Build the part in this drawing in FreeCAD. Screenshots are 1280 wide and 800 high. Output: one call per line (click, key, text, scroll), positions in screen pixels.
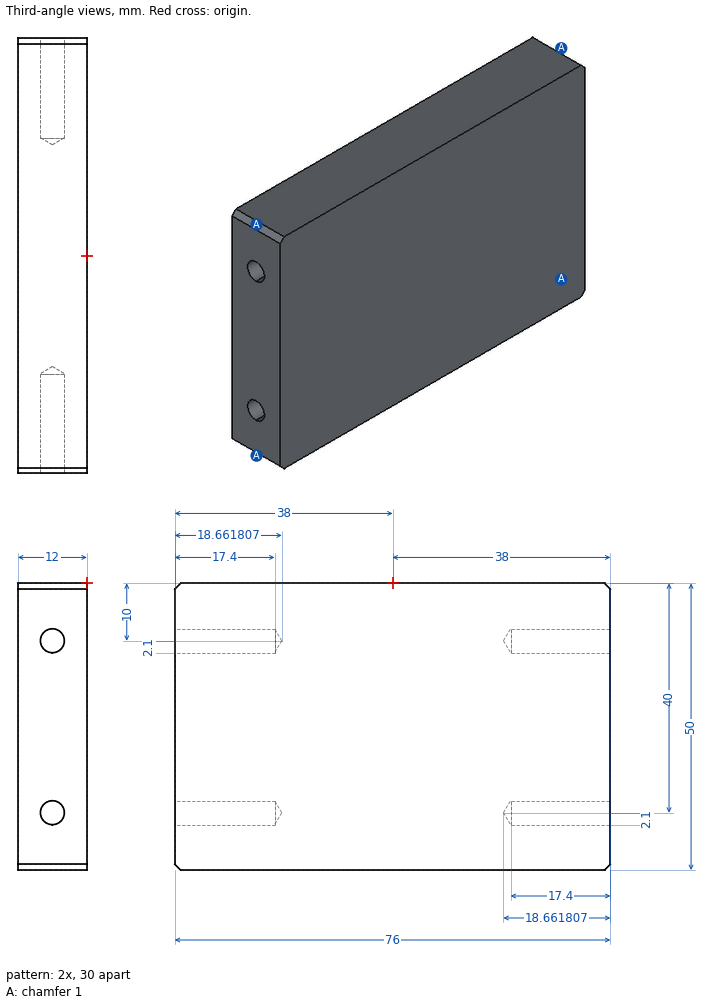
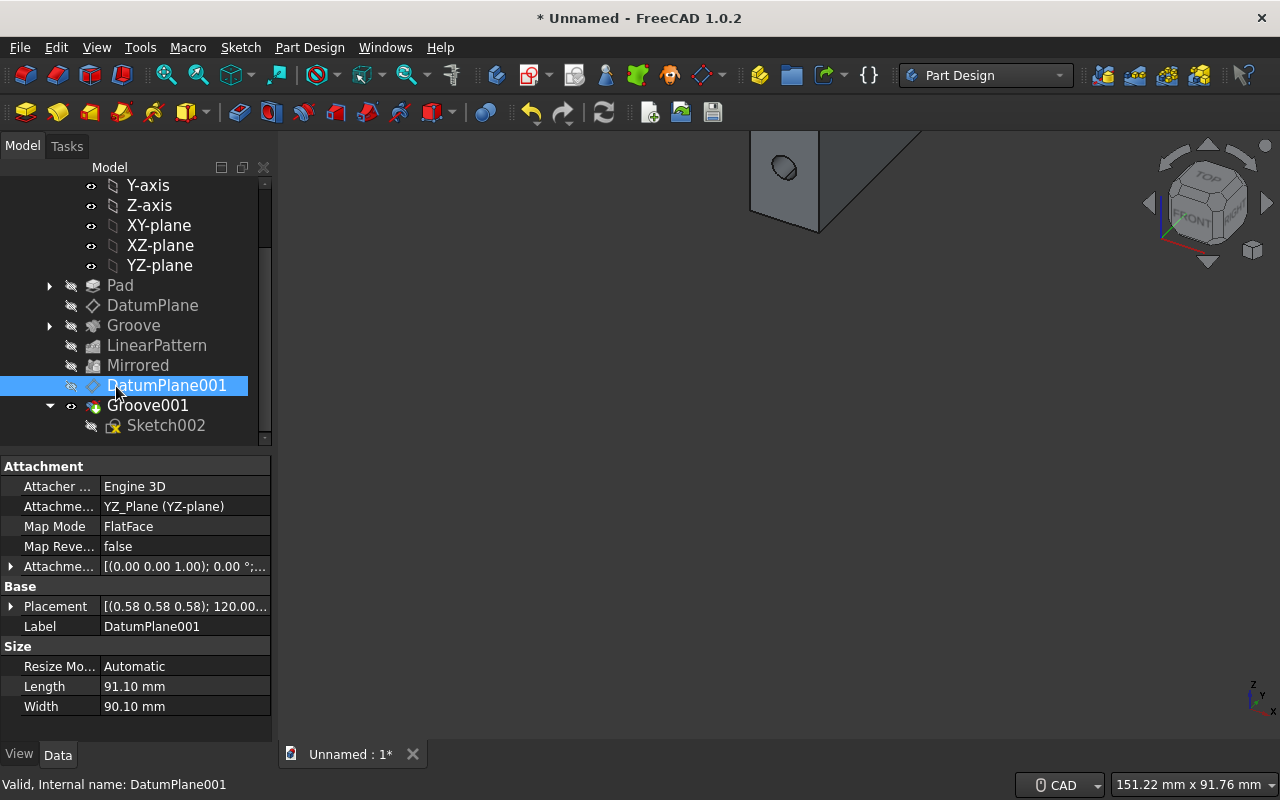
click(168, 76)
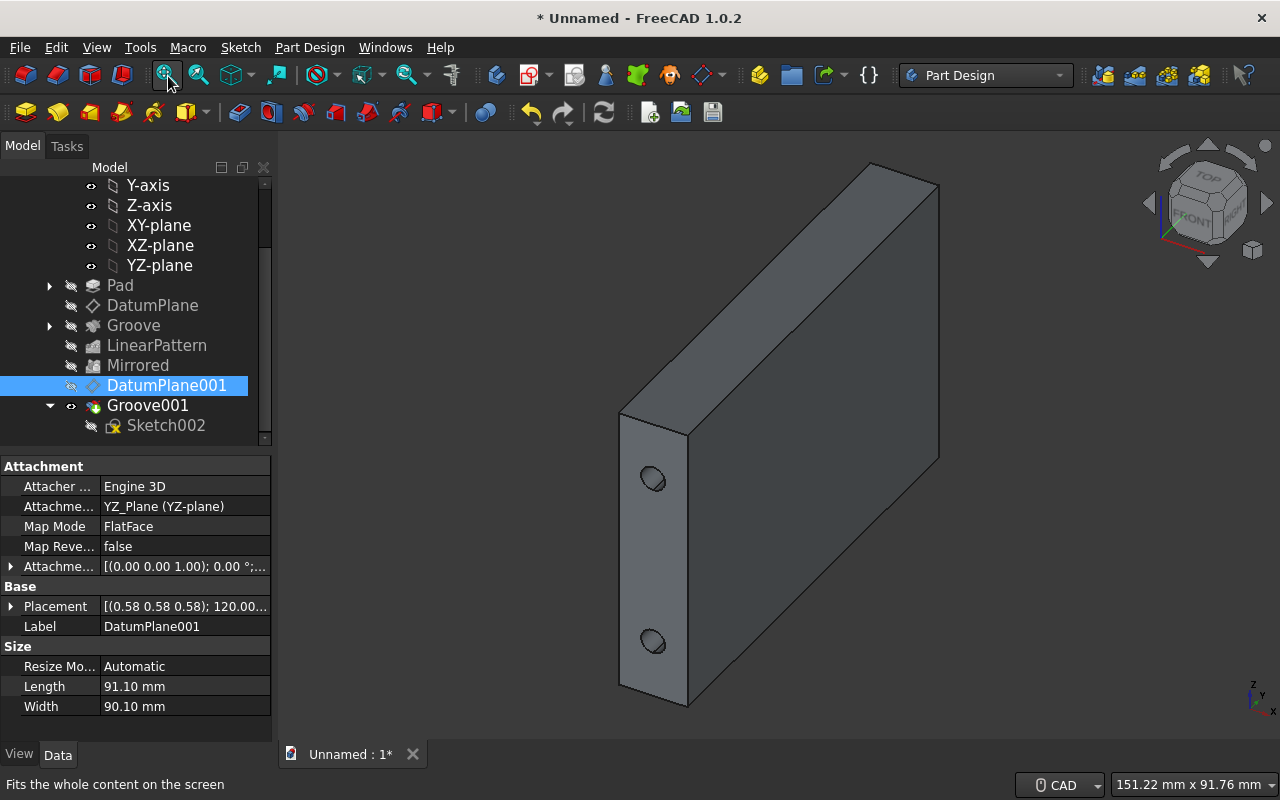
click(653, 423)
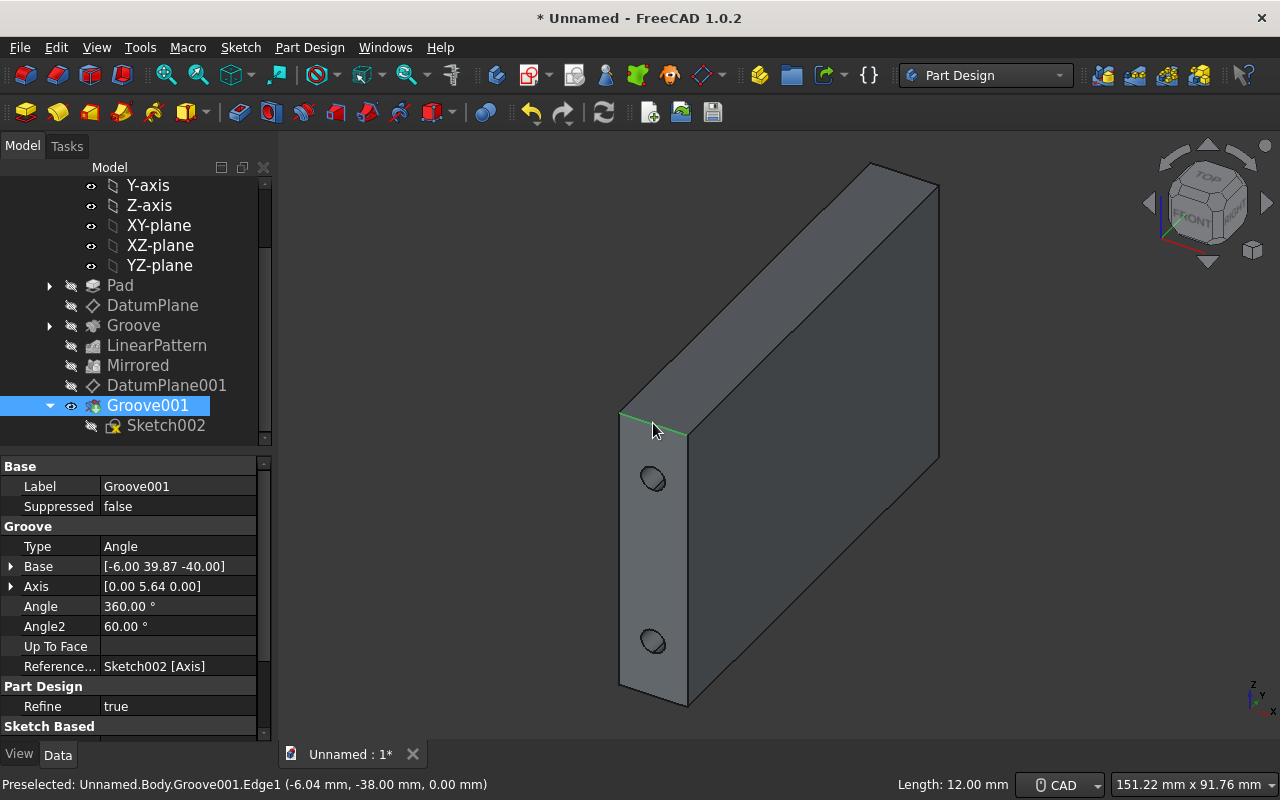
key(0)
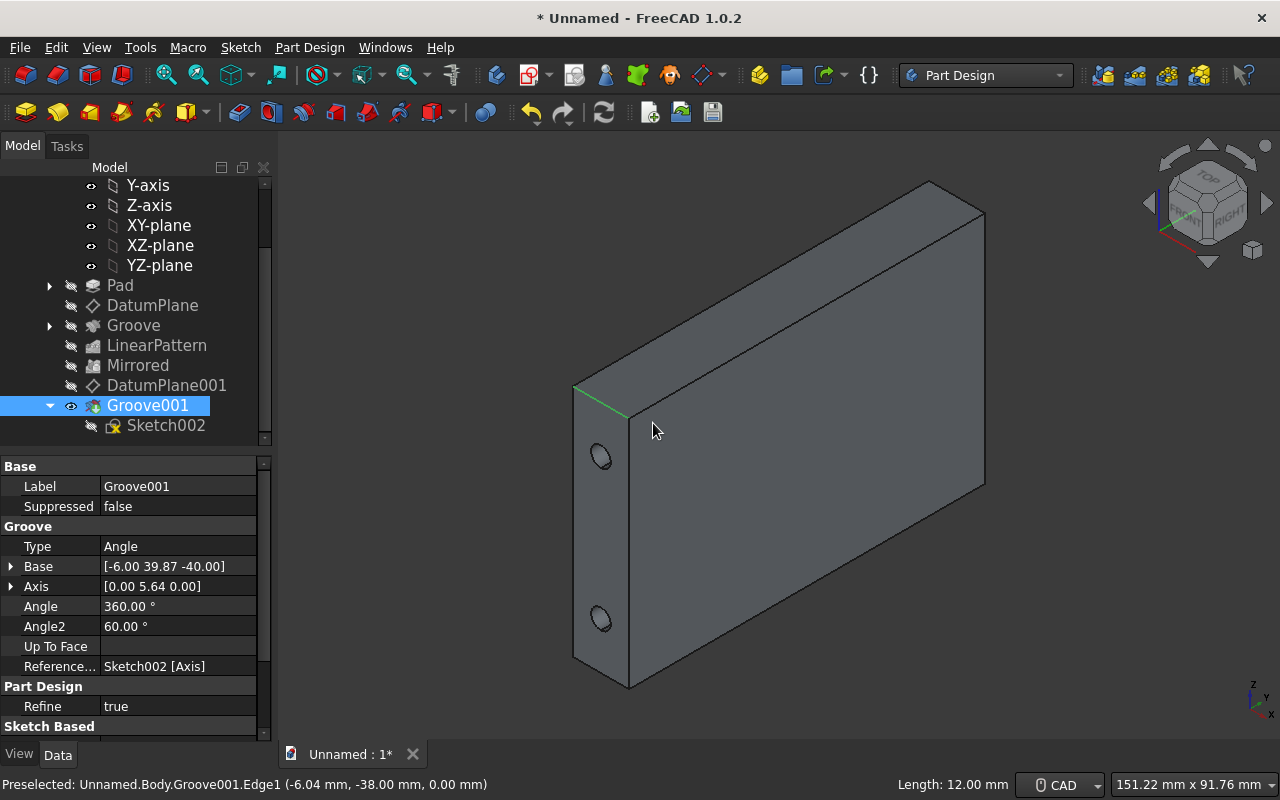
key(2)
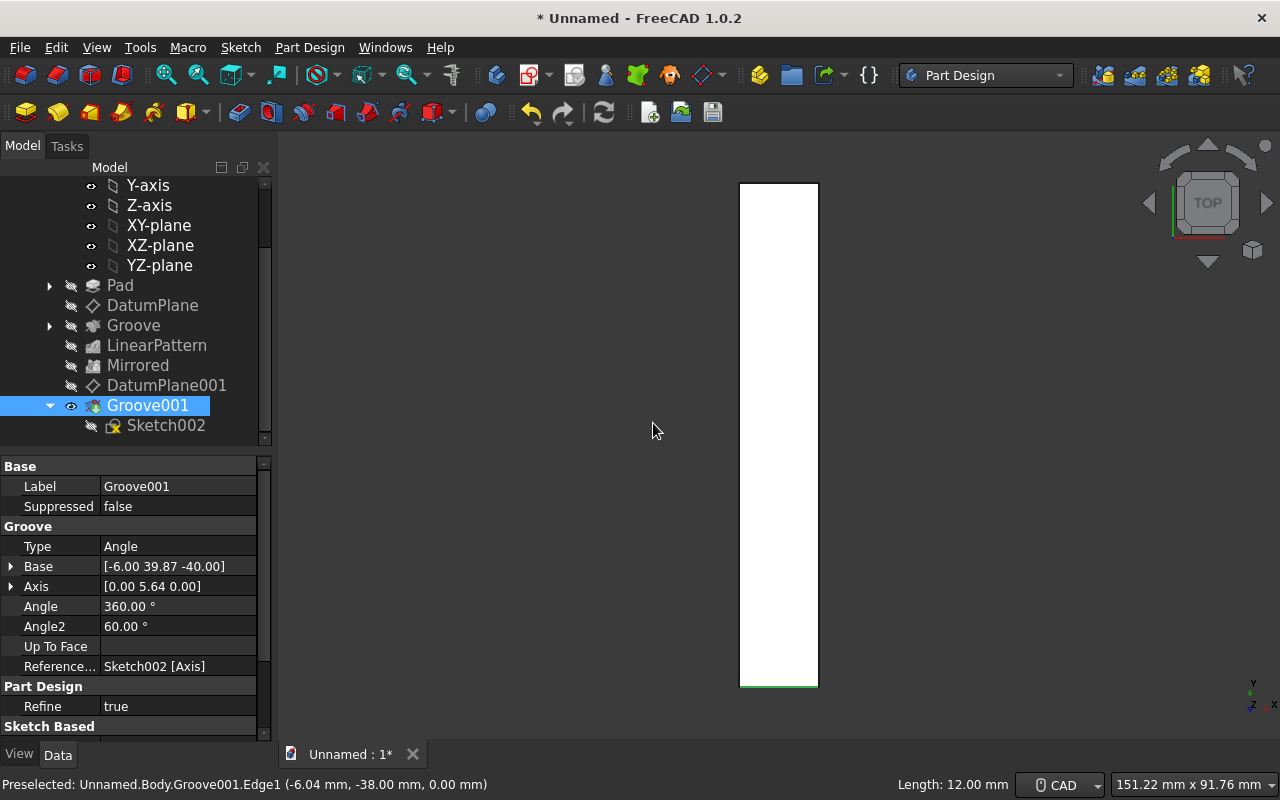
key(1)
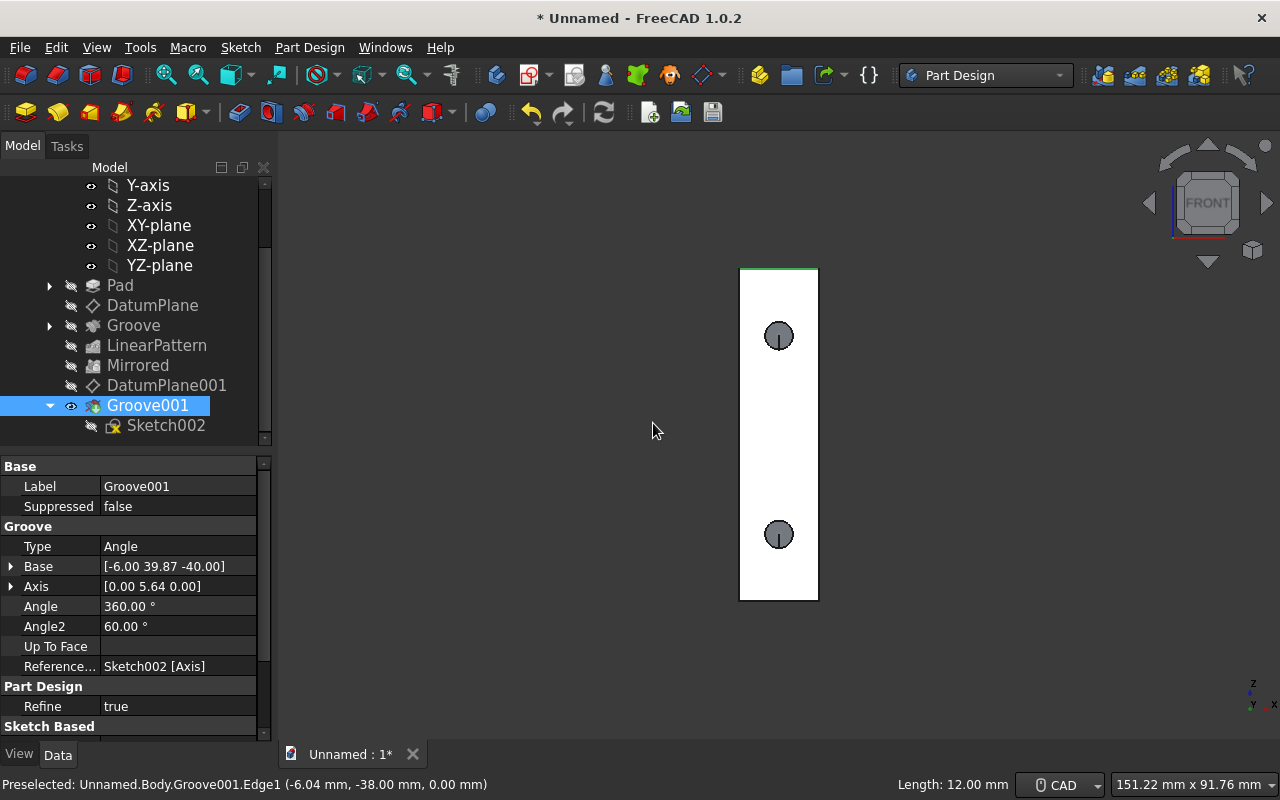
click(779, 600, ctrl)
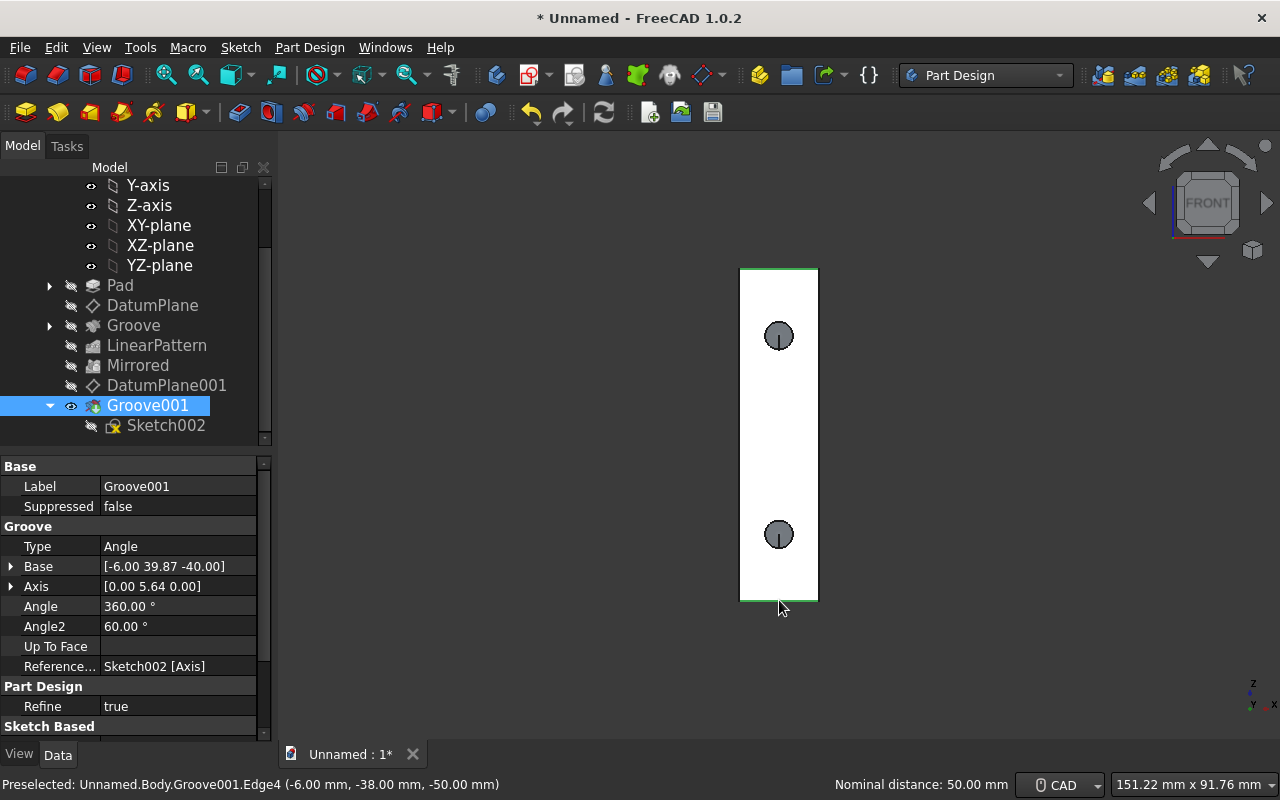
key(3)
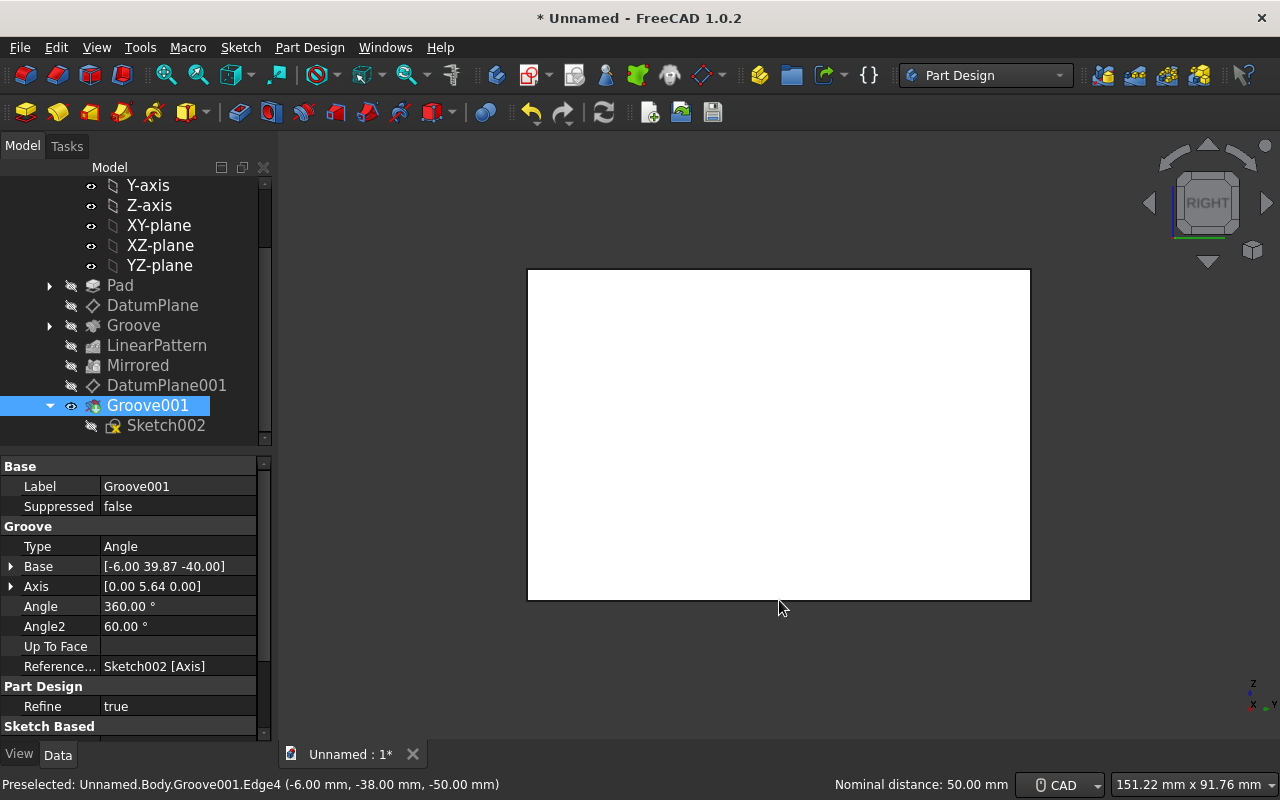
key(5)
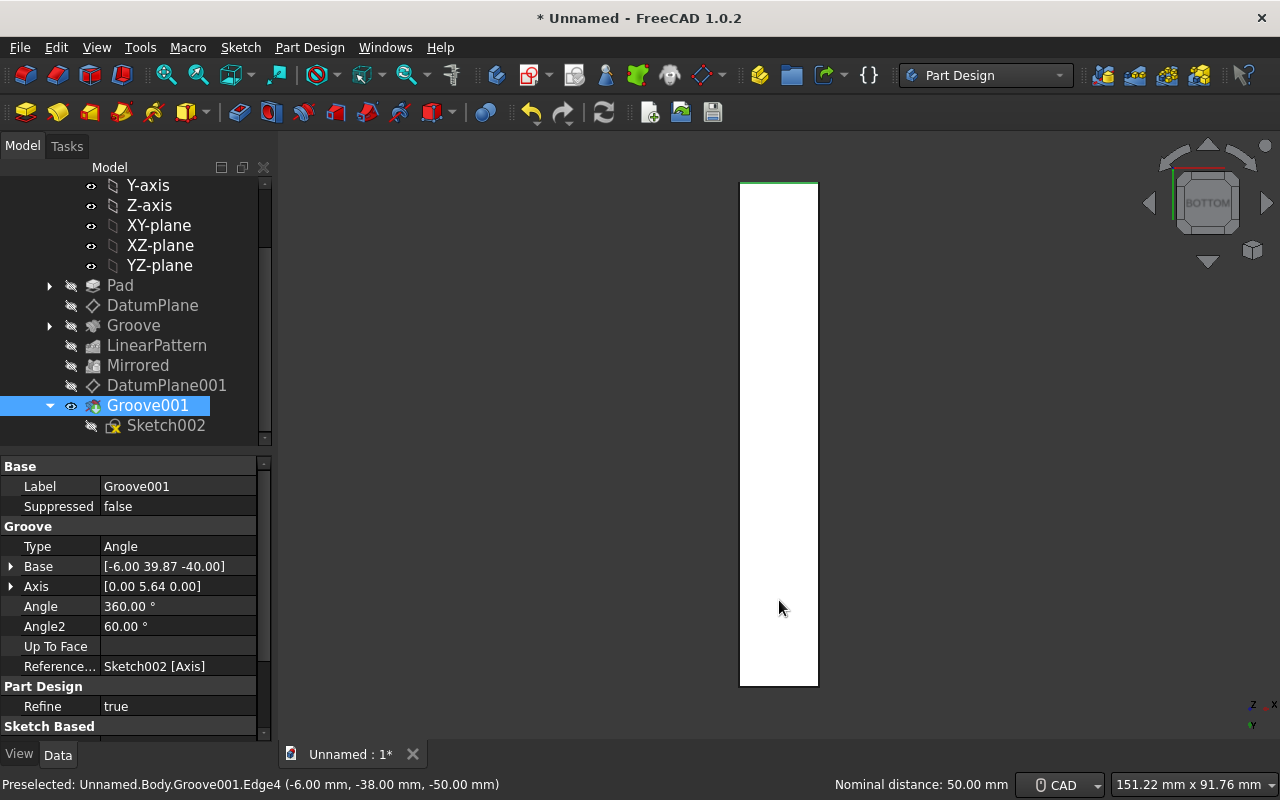
click(779, 686, ctrl)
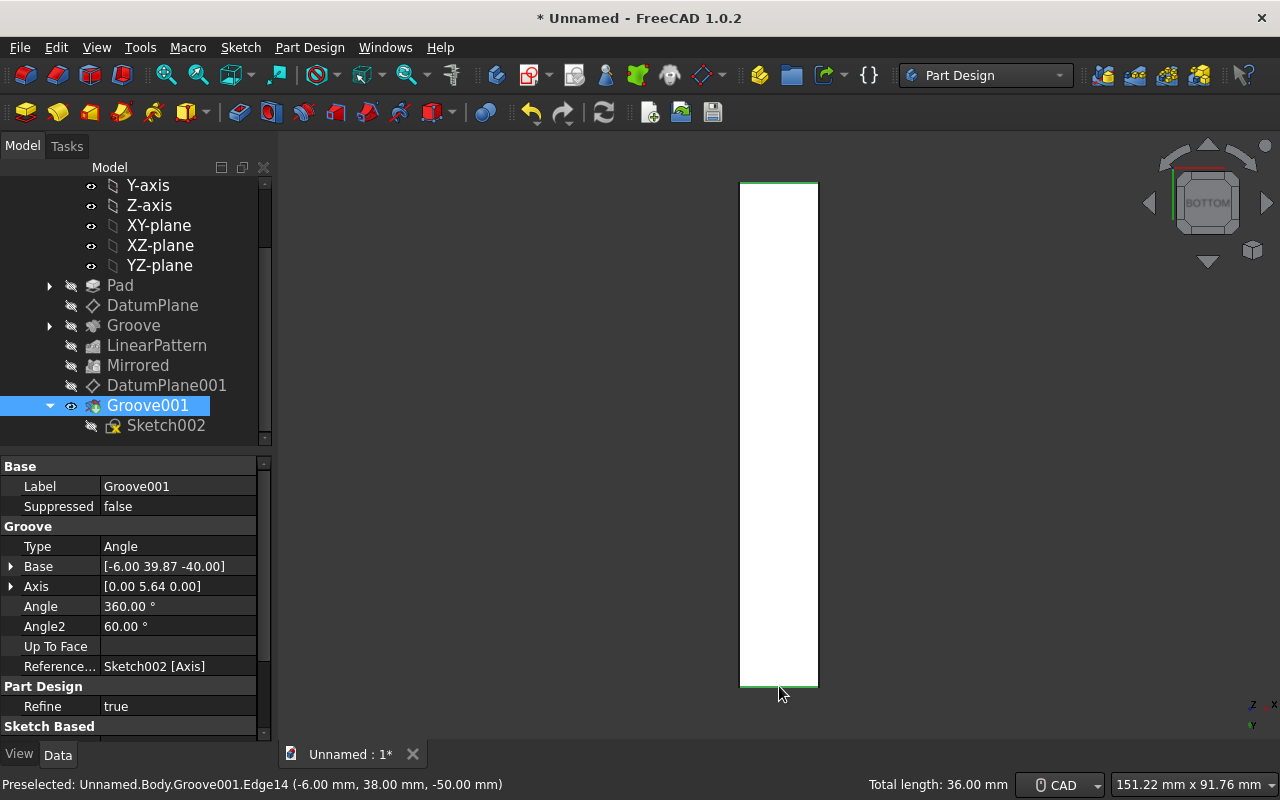
key(4)